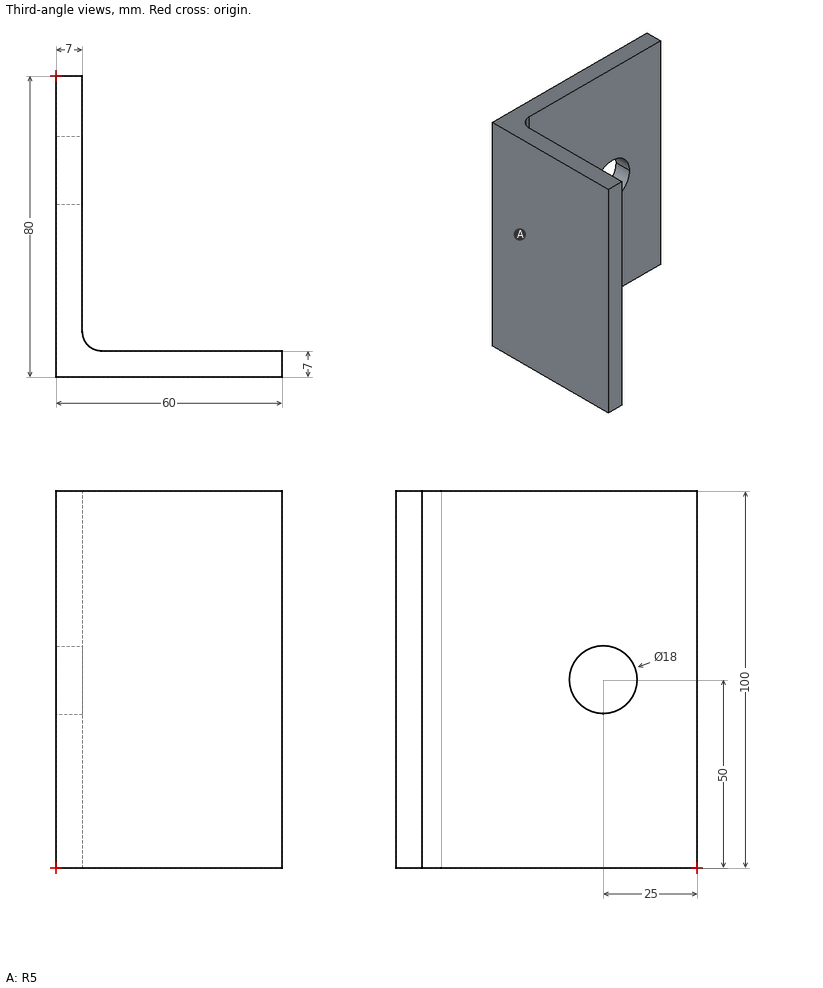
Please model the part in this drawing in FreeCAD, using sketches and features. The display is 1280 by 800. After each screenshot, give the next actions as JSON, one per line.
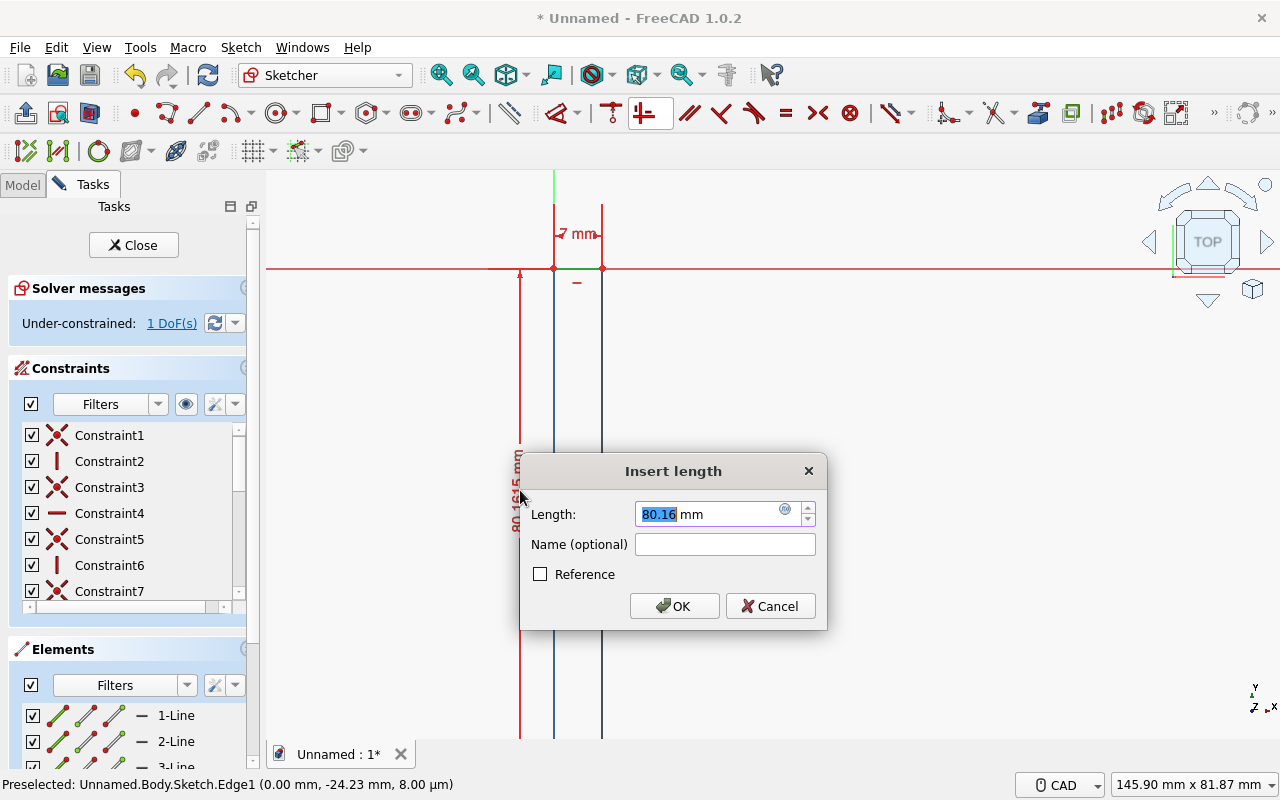
{"action": "type", "text": "80"}
{"action": "key", "text": "Return"}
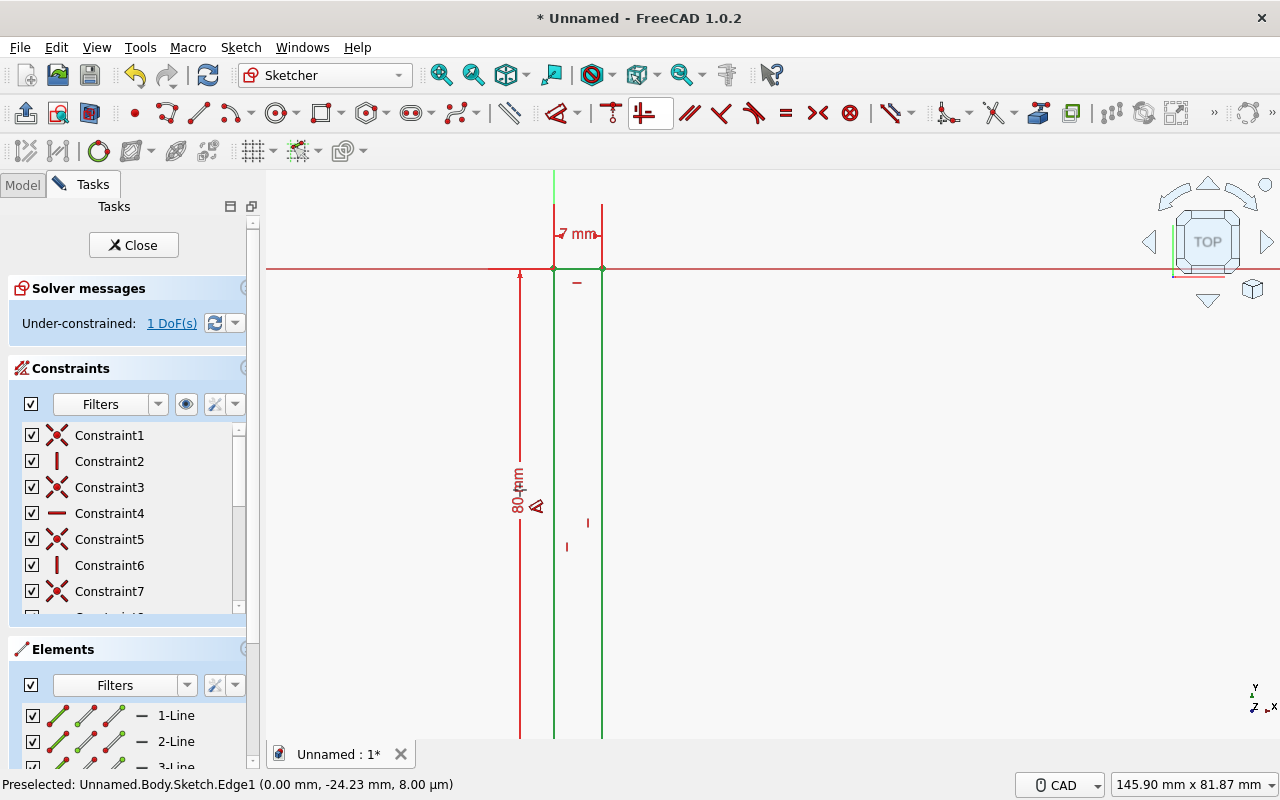
{"action": "scroll", "coordinate": [587, 267], "scroll_direction": "down", "scroll_amount": 2}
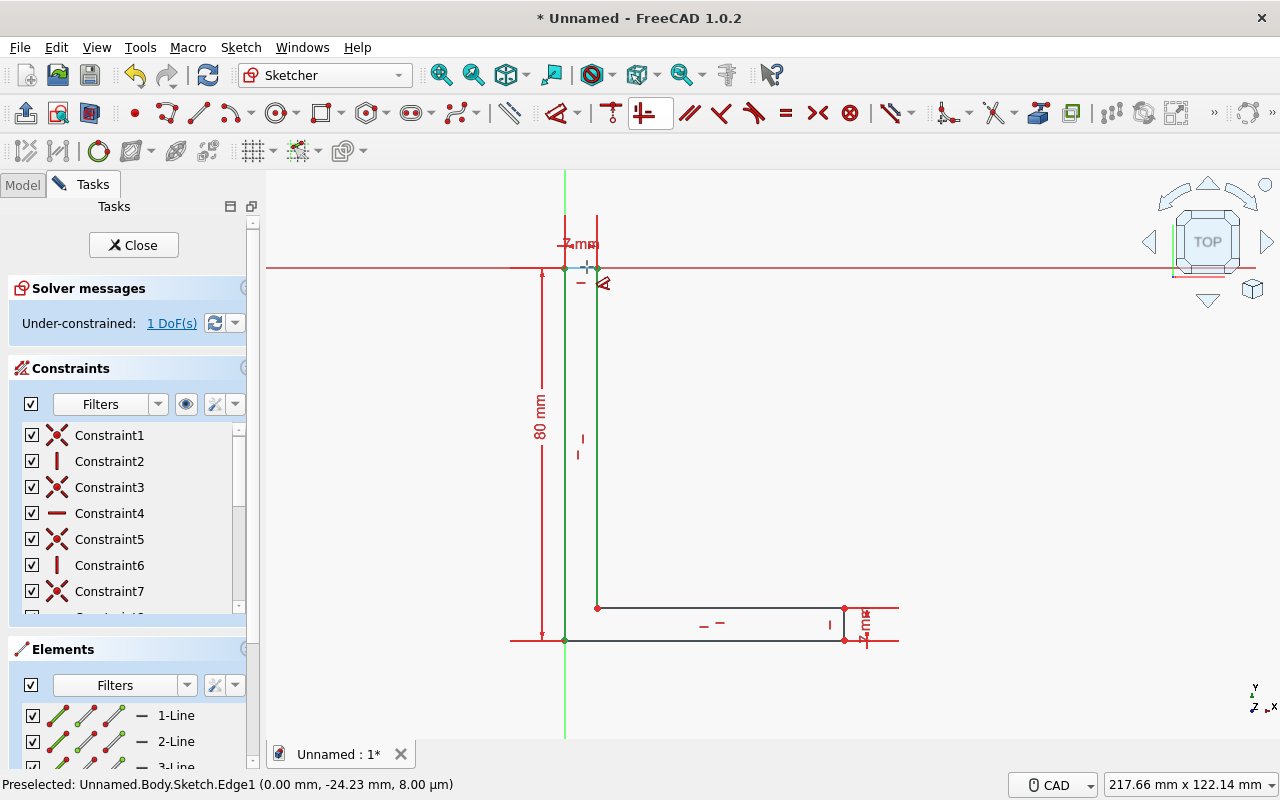
{"action": "left_click", "coordinate": [649, 641]}
{"action": "left_click", "coordinate": [705, 675]}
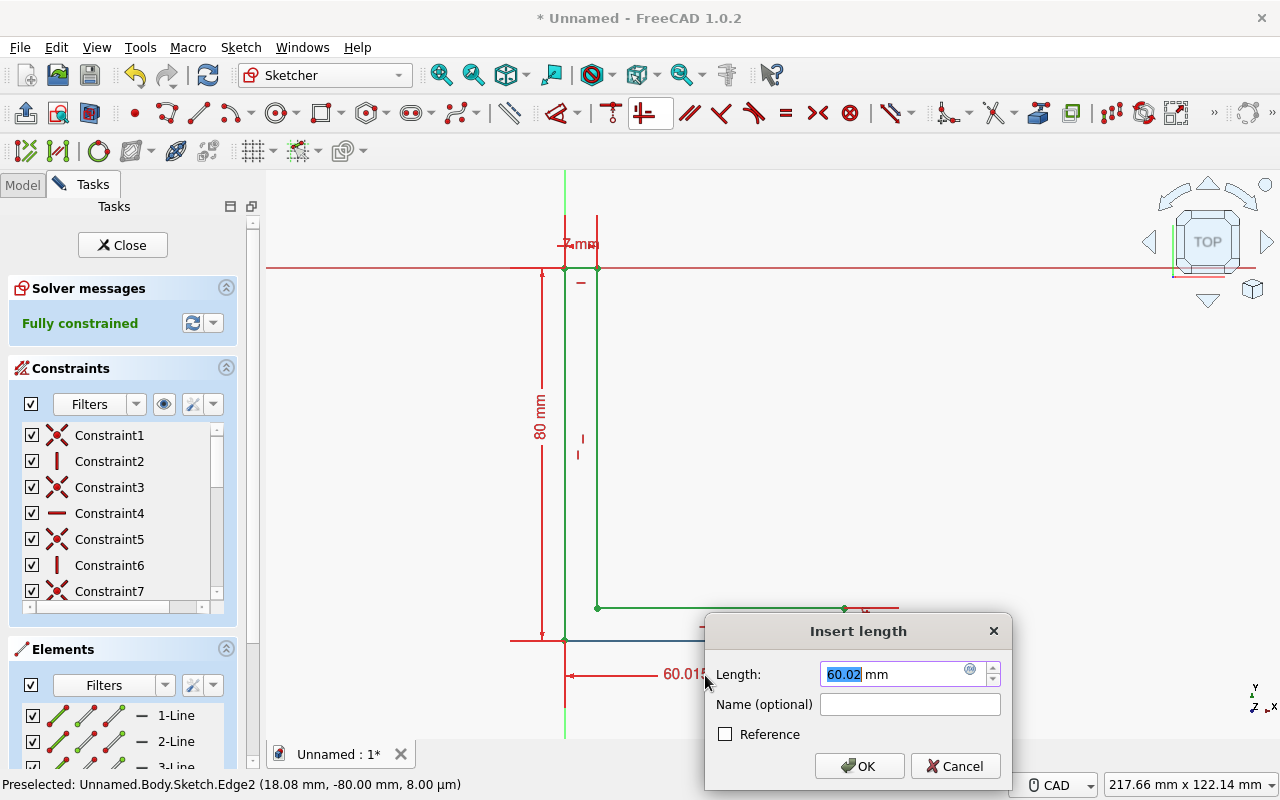
{"action": "type", "text": "60"}
{"action": "key", "text": "Return"}
{"action": "key", "text": "Escape"}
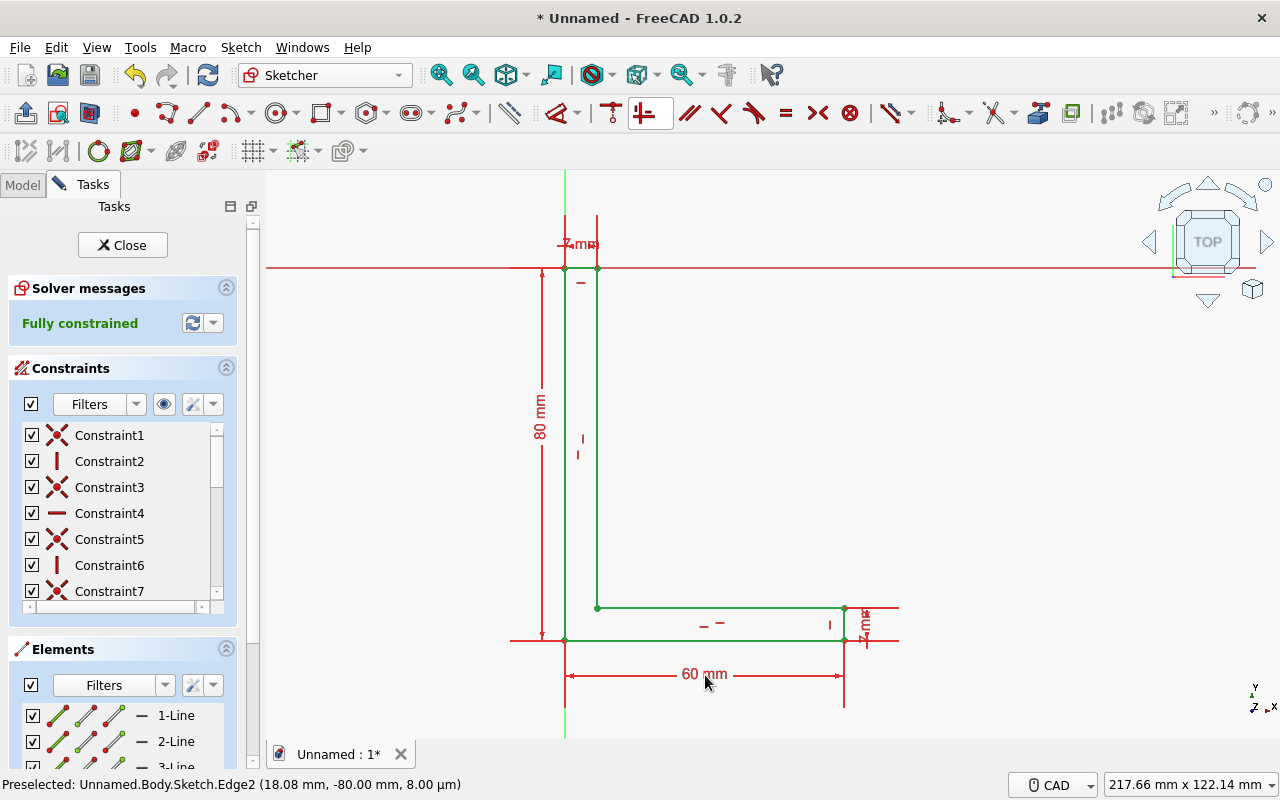
{"action": "left_click", "coordinate": [123, 245]}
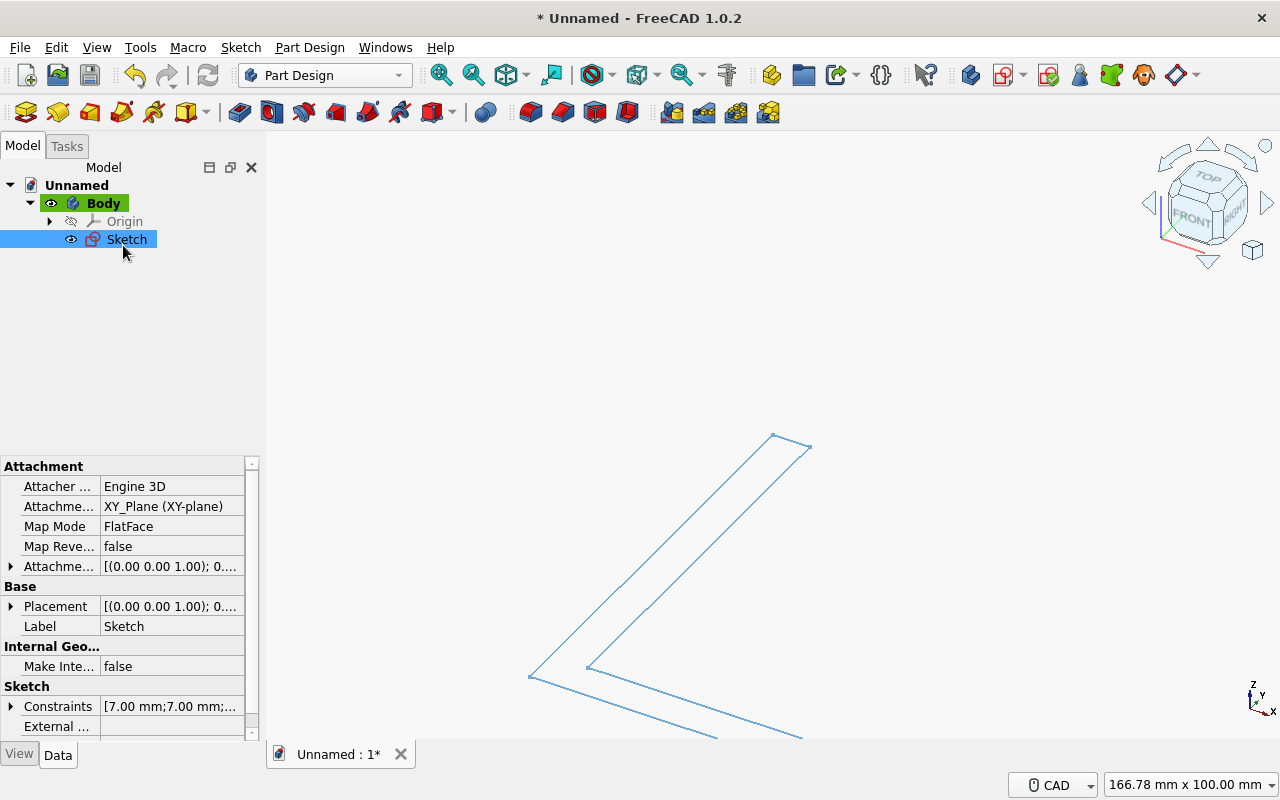
{"action": "left_click", "coordinate": [26, 112]}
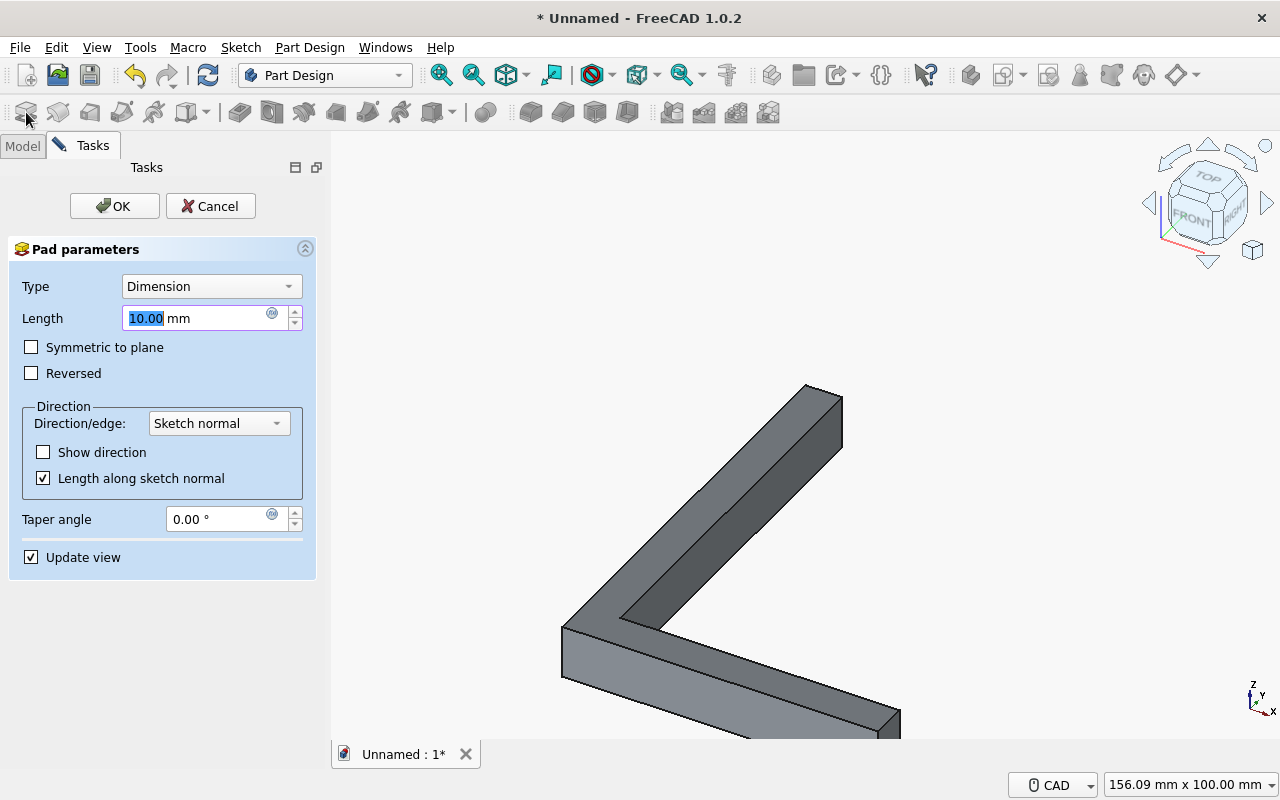
{"action": "type", "text": "100"}
{"action": "key", "text": "Tab"}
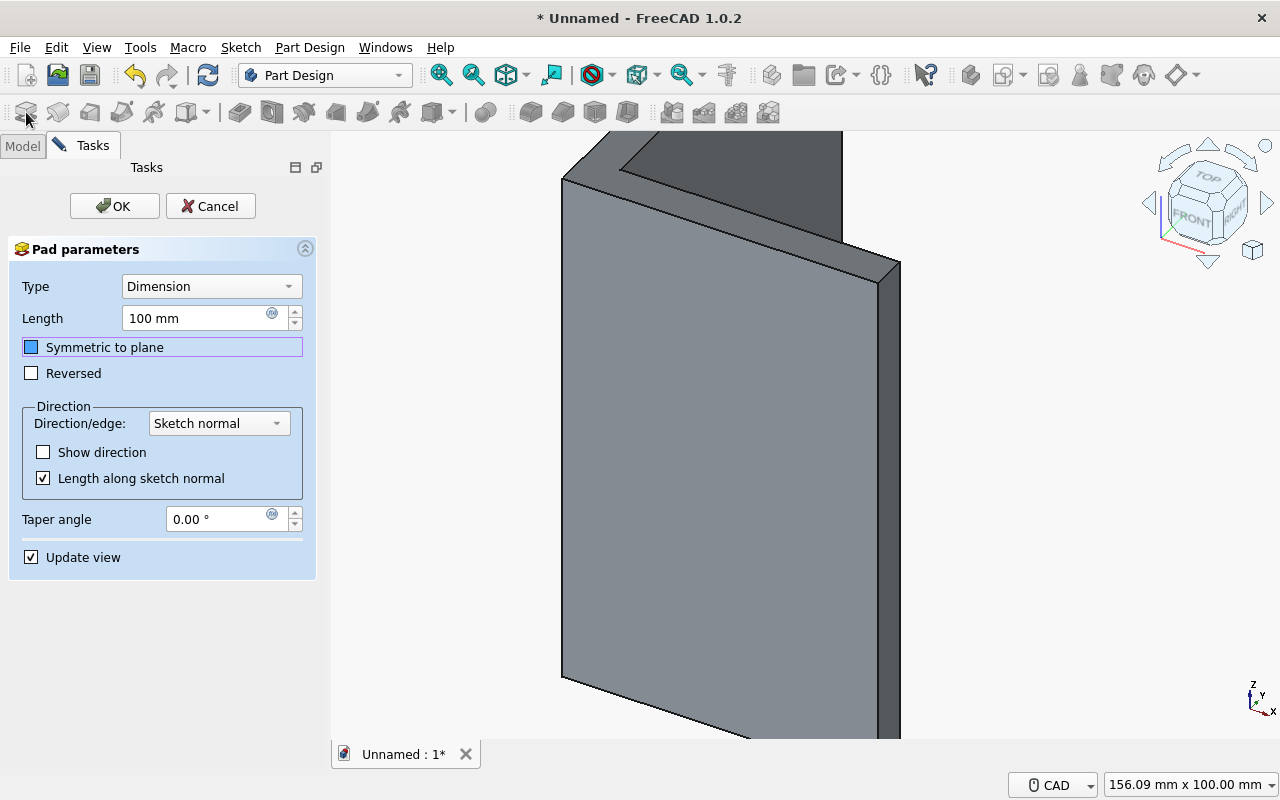
{"action": "left_click", "coordinate": [115, 206]}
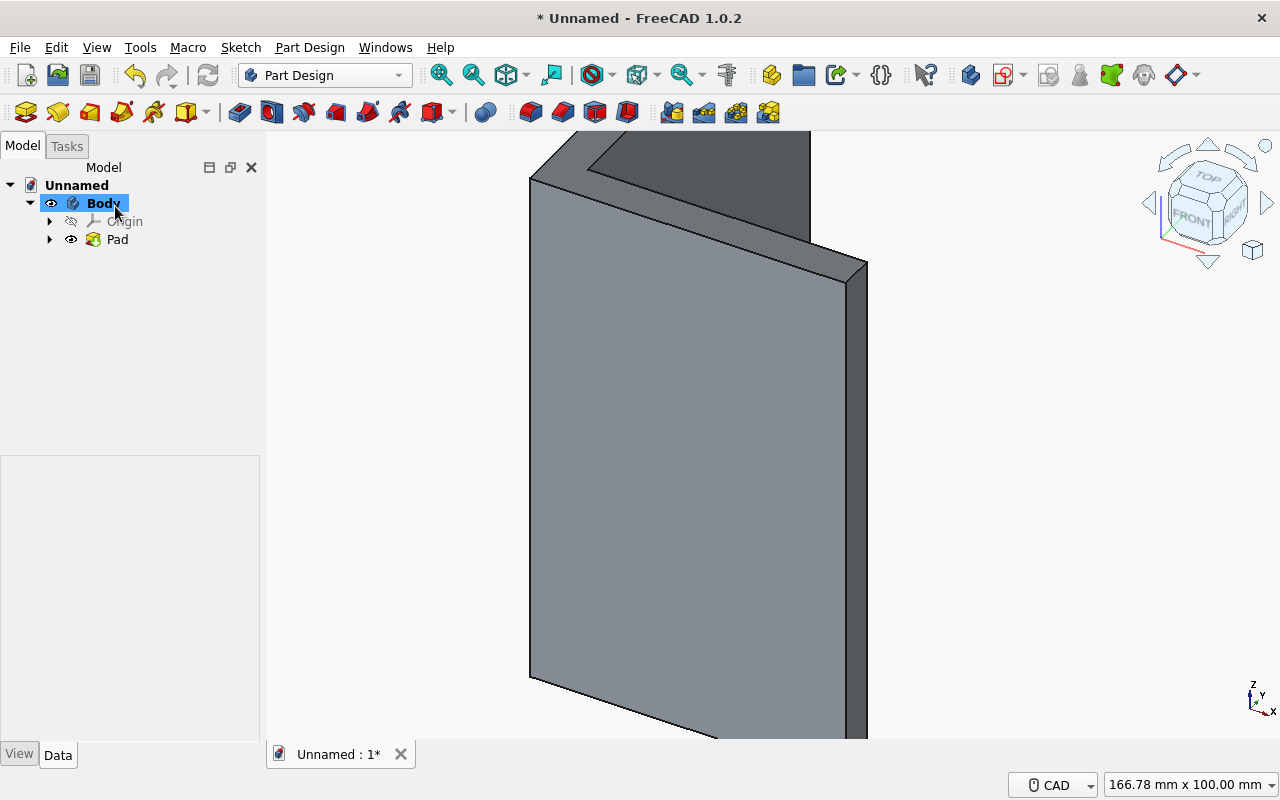
{"action": "key", "text": "v f"}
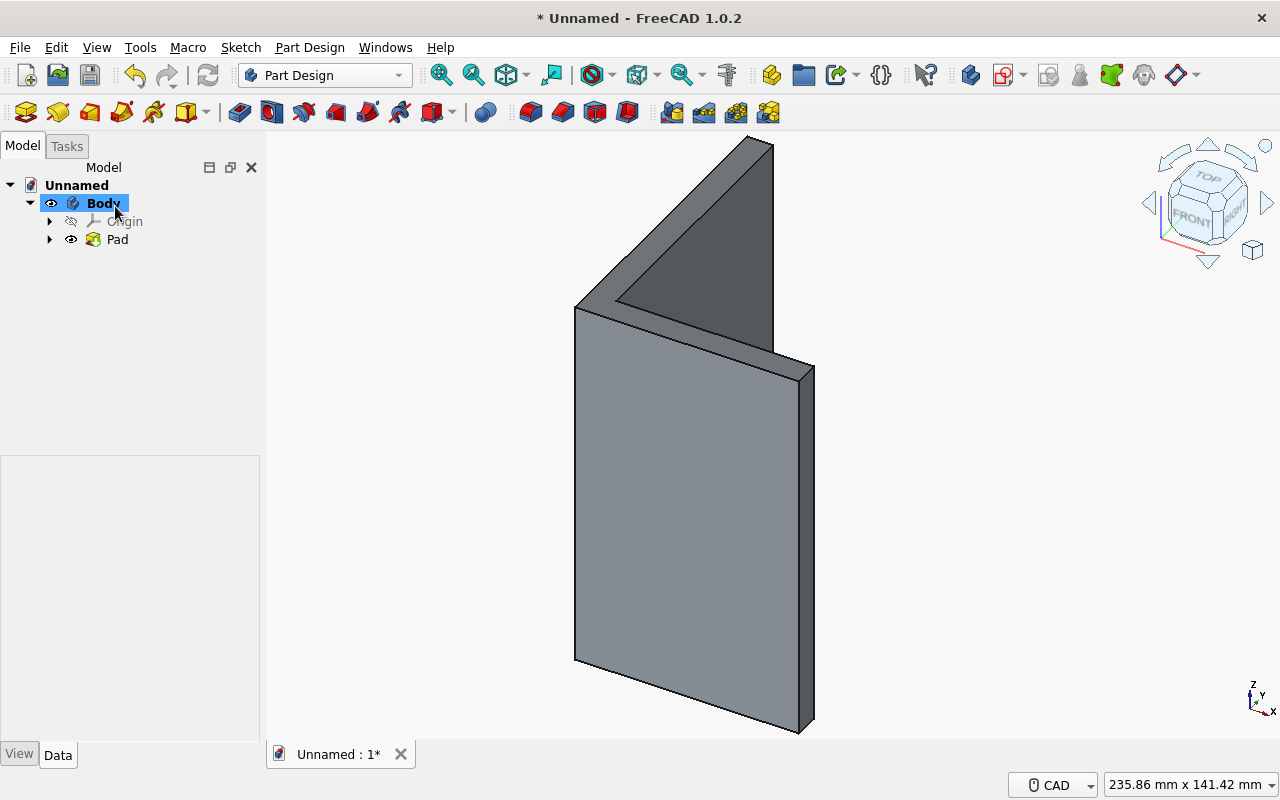
{"action": "key", "text": "0"}